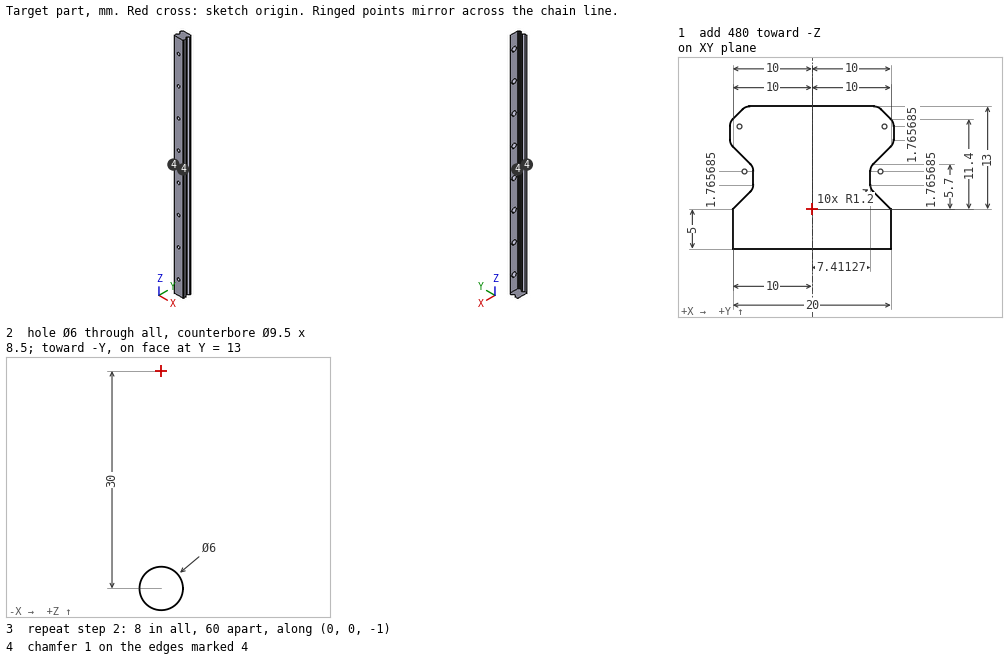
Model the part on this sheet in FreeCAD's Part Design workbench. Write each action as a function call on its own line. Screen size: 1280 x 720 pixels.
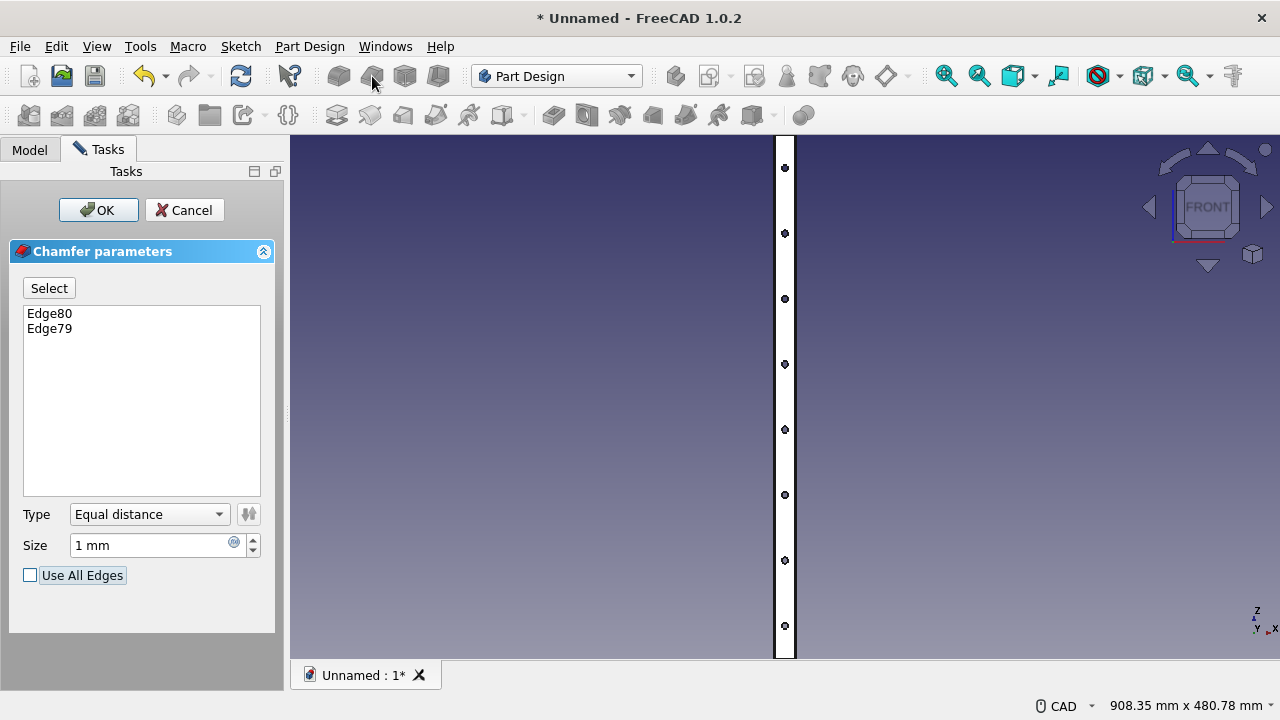
click(99, 210)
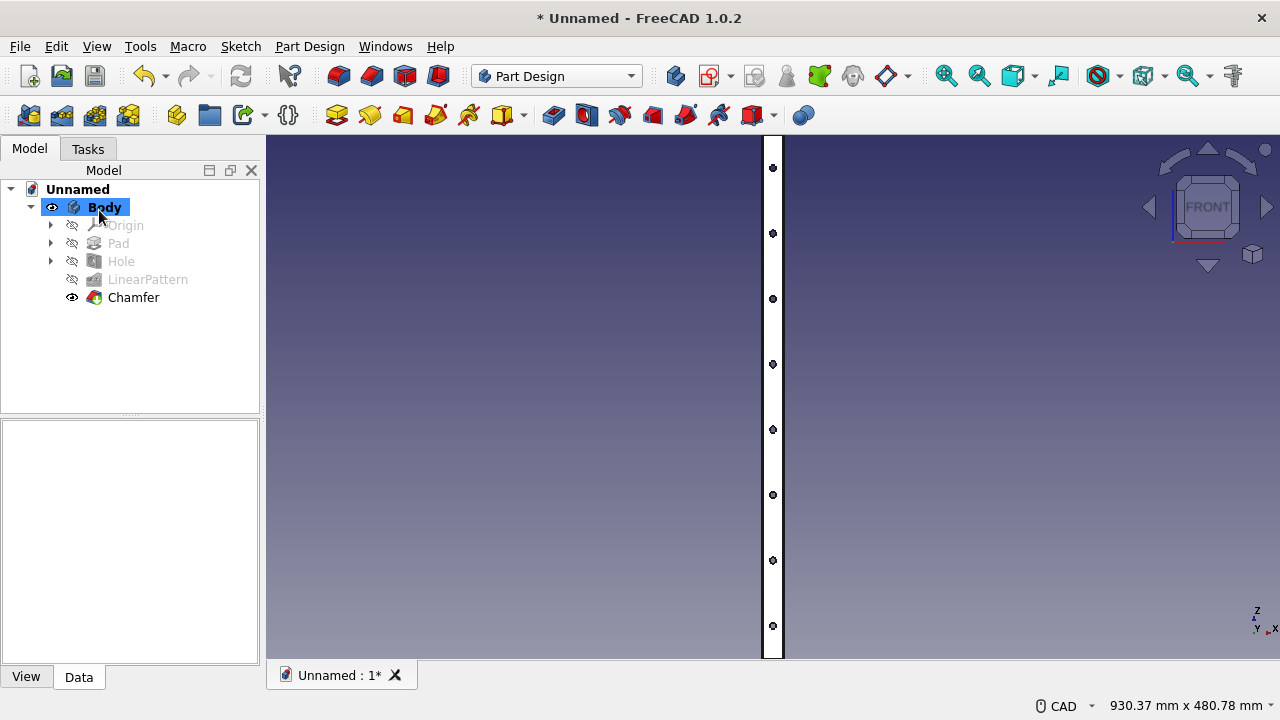
key(0)